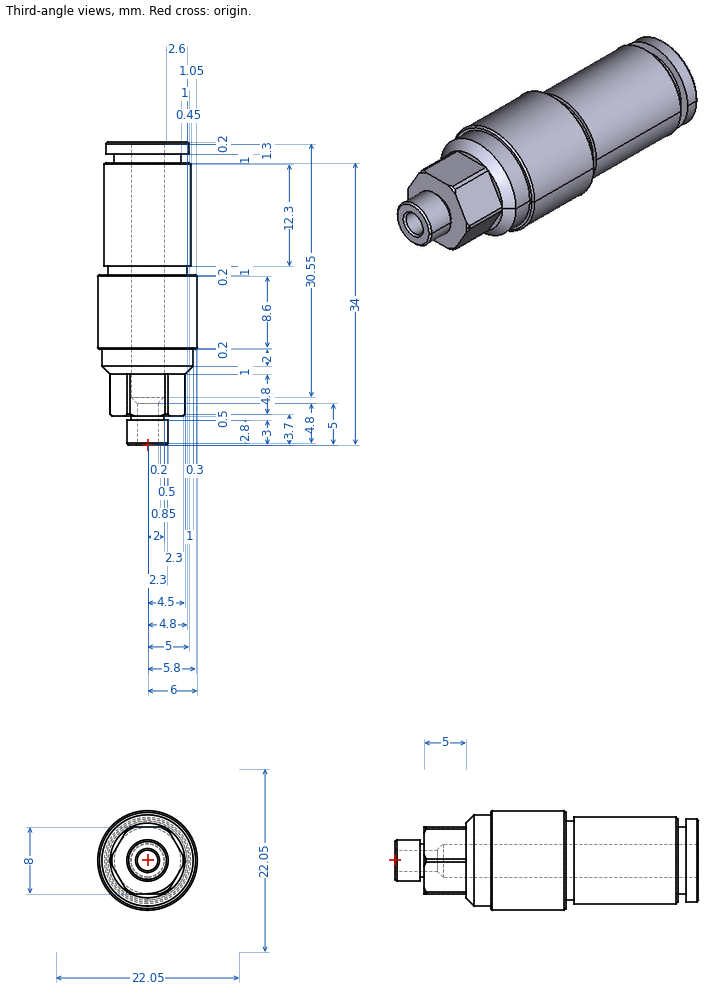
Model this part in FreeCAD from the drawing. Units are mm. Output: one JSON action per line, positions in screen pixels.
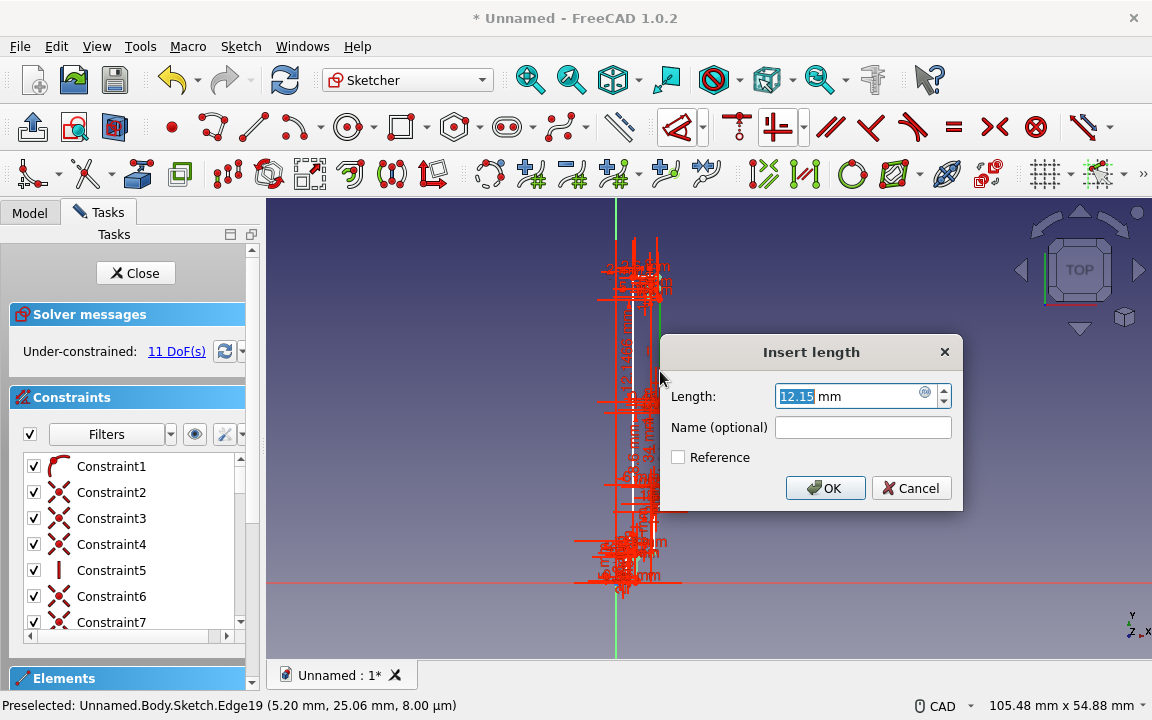
{"action": "type", "text": "12.3"}
{"action": "key", "text": "Return"}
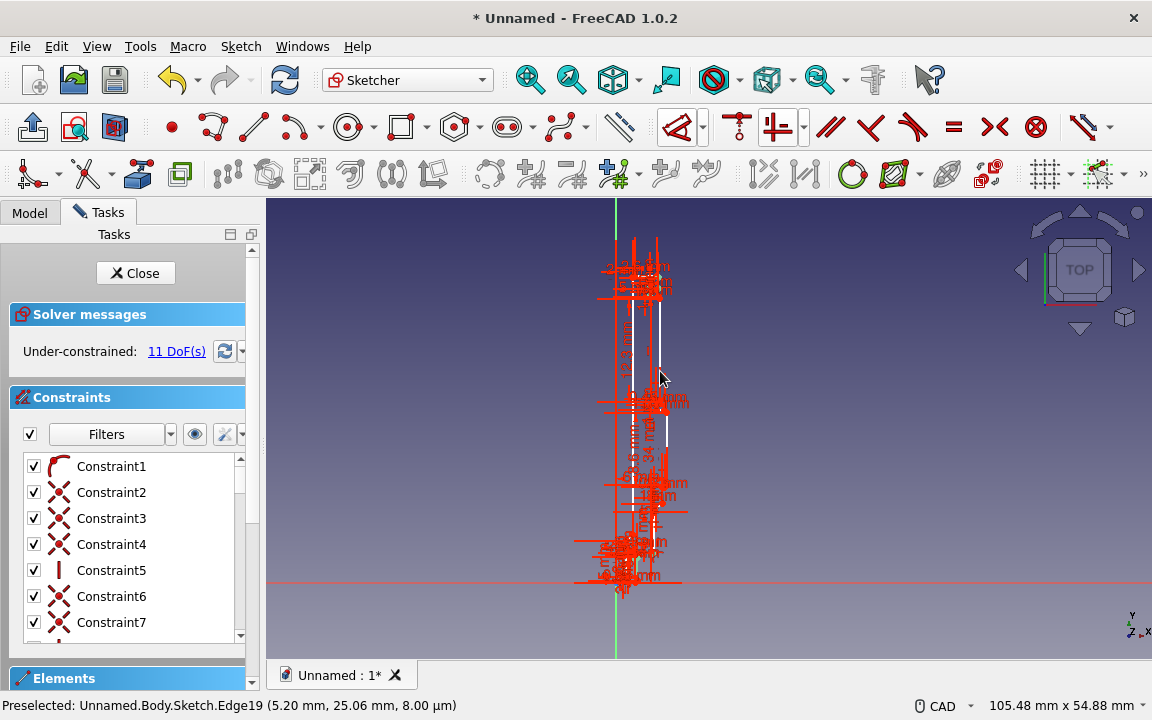
{"action": "scroll", "coordinate": [635, 583], "scroll_direction": "up", "scroll_amount": 9}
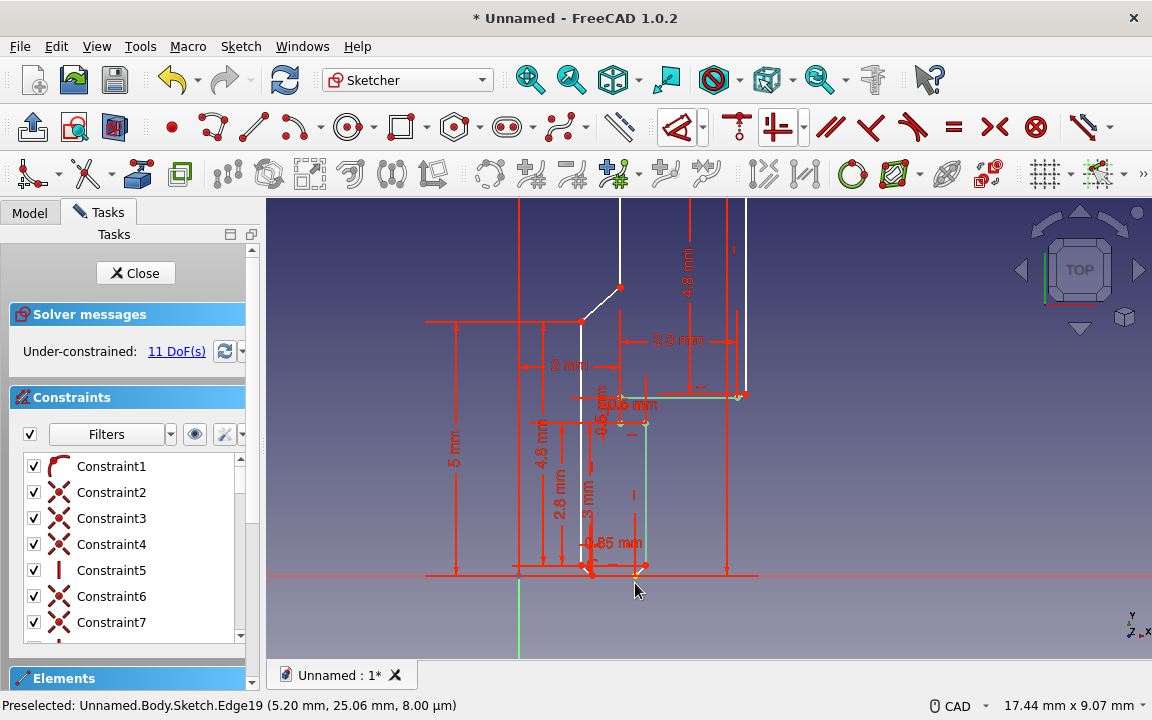
{"action": "left_click", "coordinate": [635, 576]}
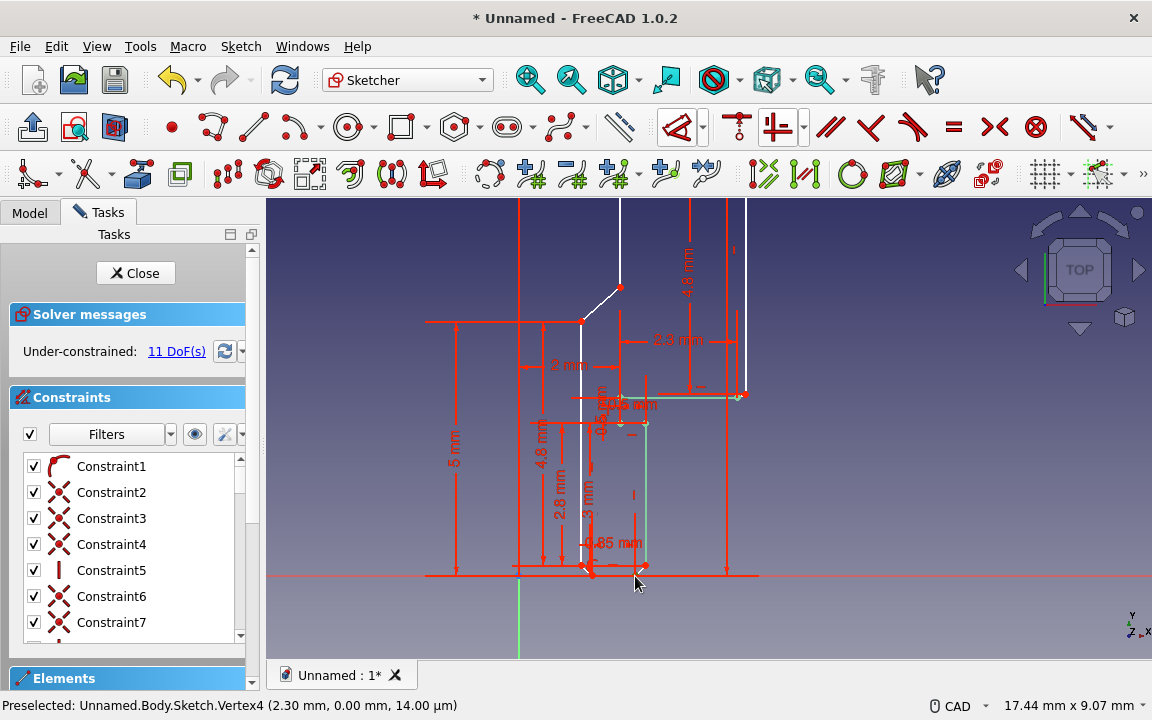
{"action": "left_click", "coordinate": [702, 128]}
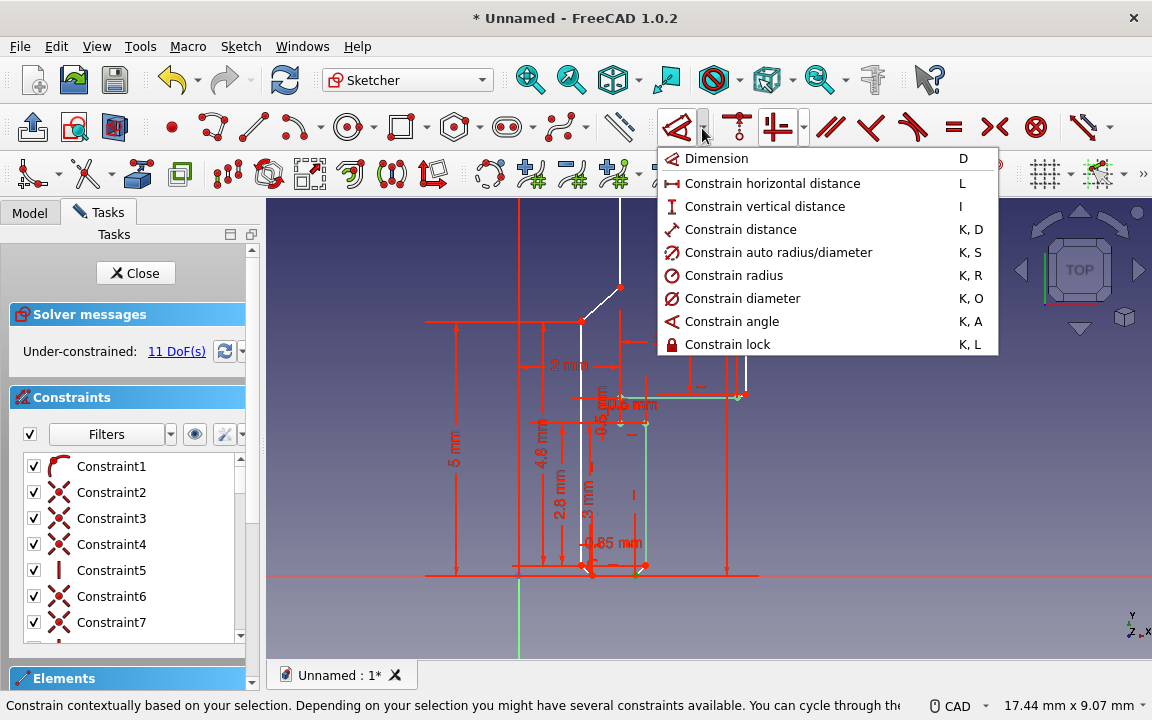
{"action": "left_click", "coordinate": [828, 184]}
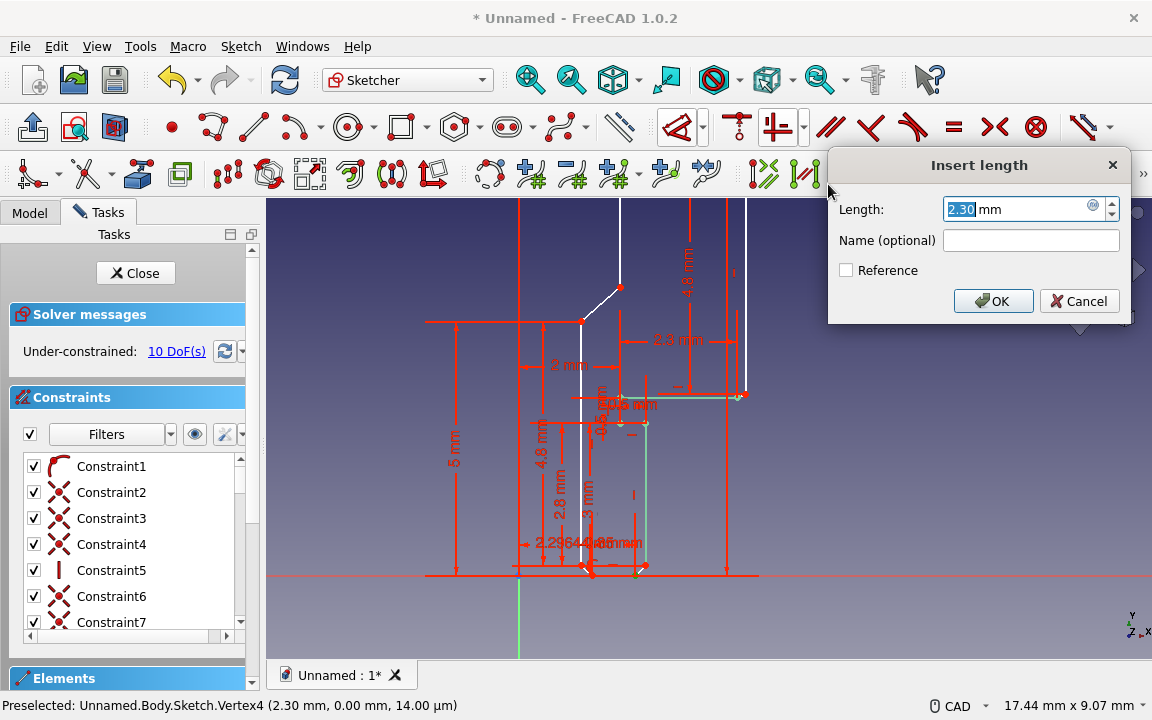
{"action": "type", "text": "2.3"}
{"action": "key", "text": "Return"}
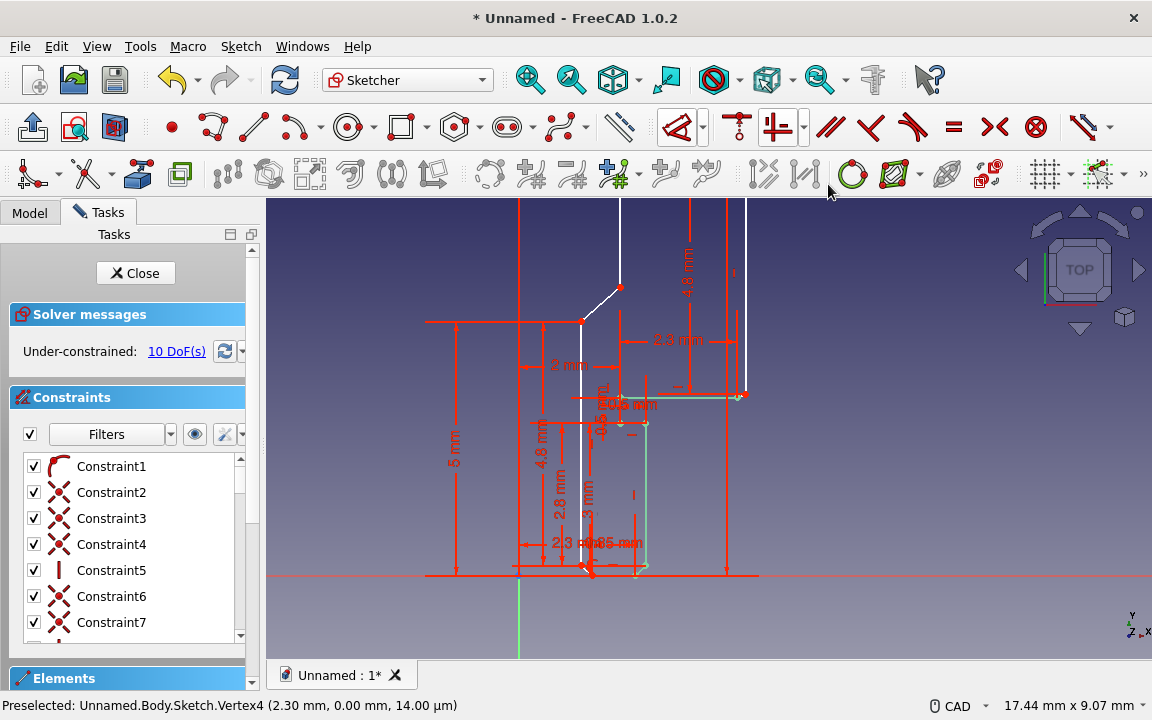
{"action": "scroll", "coordinate": [746, 394], "scroll_direction": "up", "scroll_amount": 2}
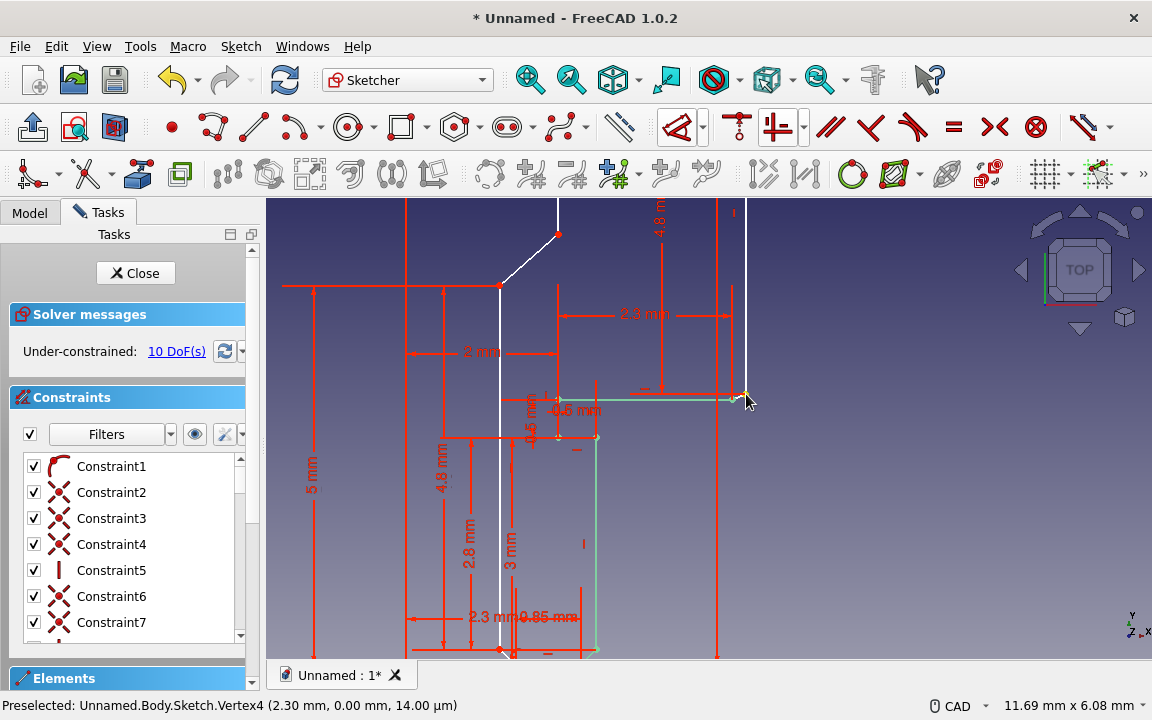
{"action": "left_click", "coordinate": [746, 394]}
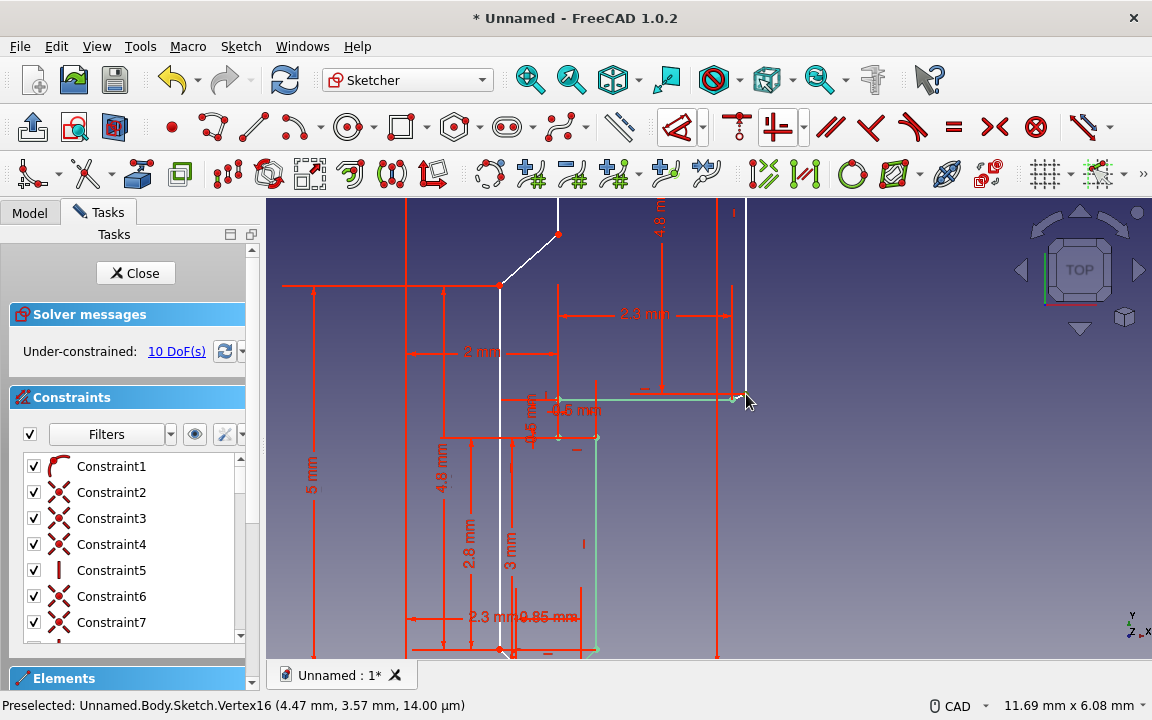
{"action": "left_click", "coordinate": [702, 128]}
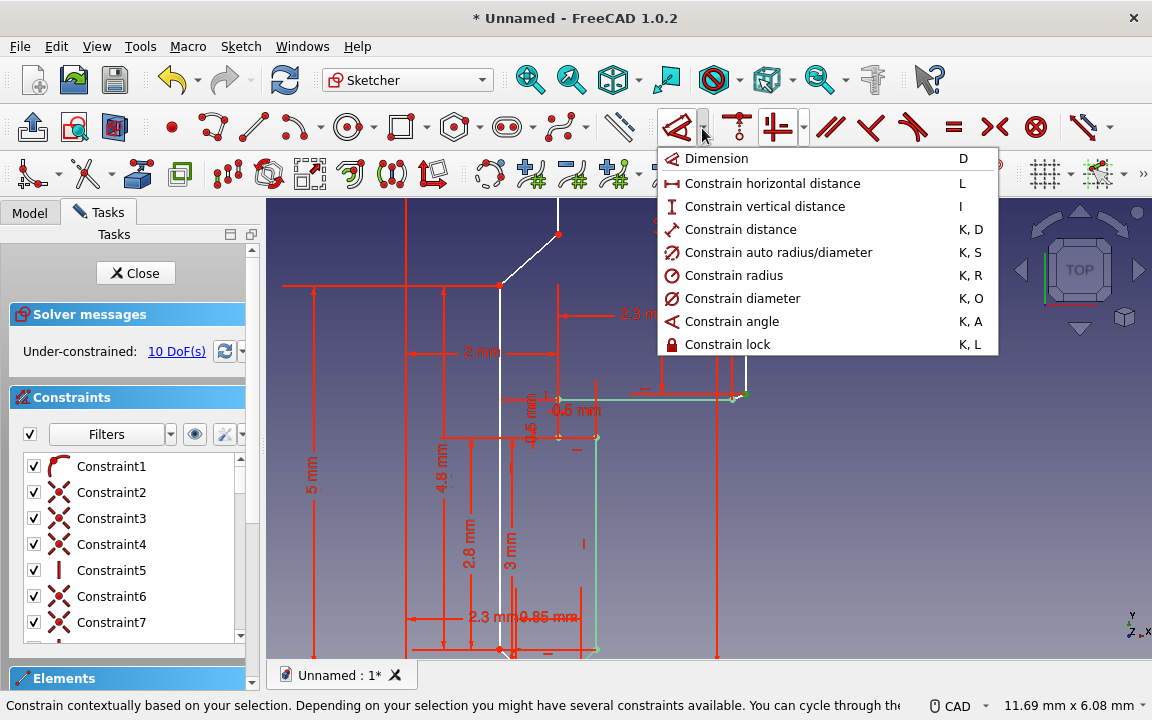
{"action": "left_click", "coordinate": [828, 184]}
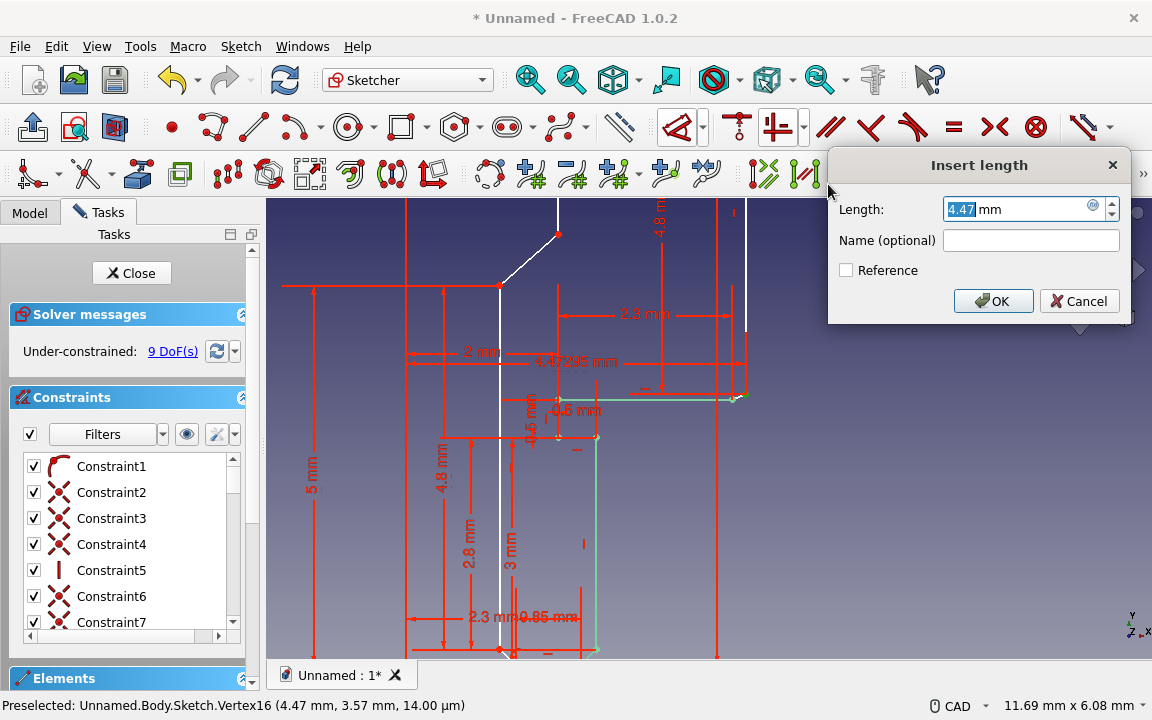
{"action": "type", "text": "4.5"}
{"action": "key", "text": "Return"}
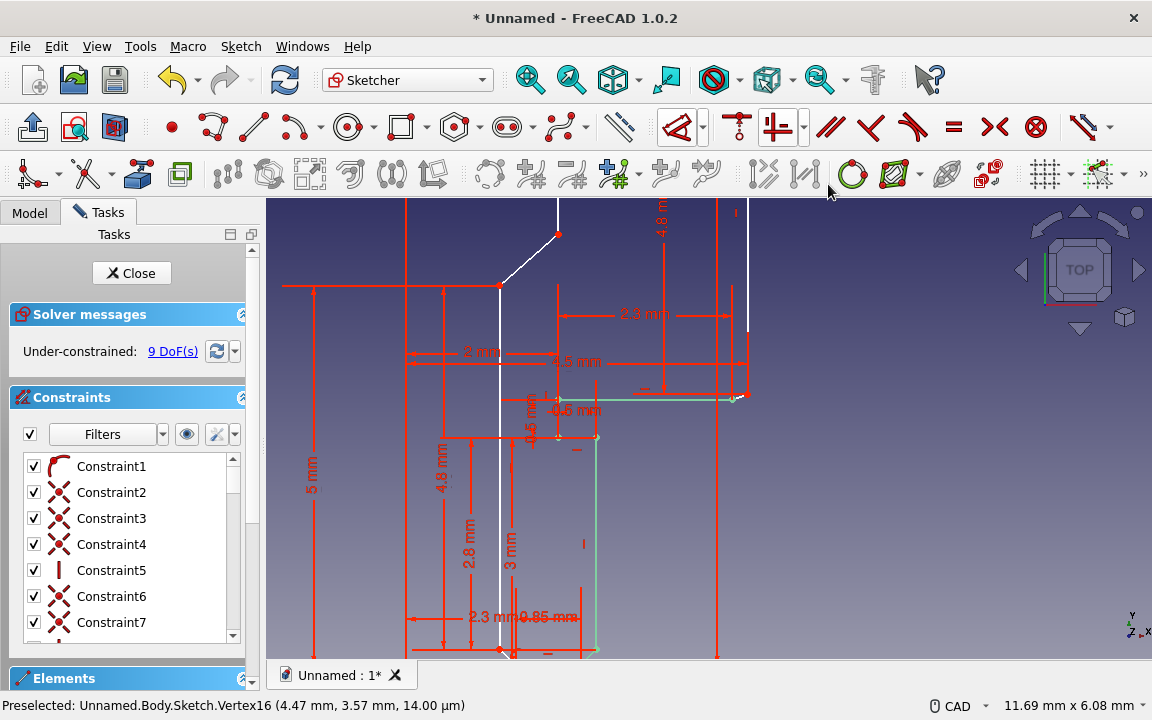
{"action": "left_click", "coordinate": [748, 394]}